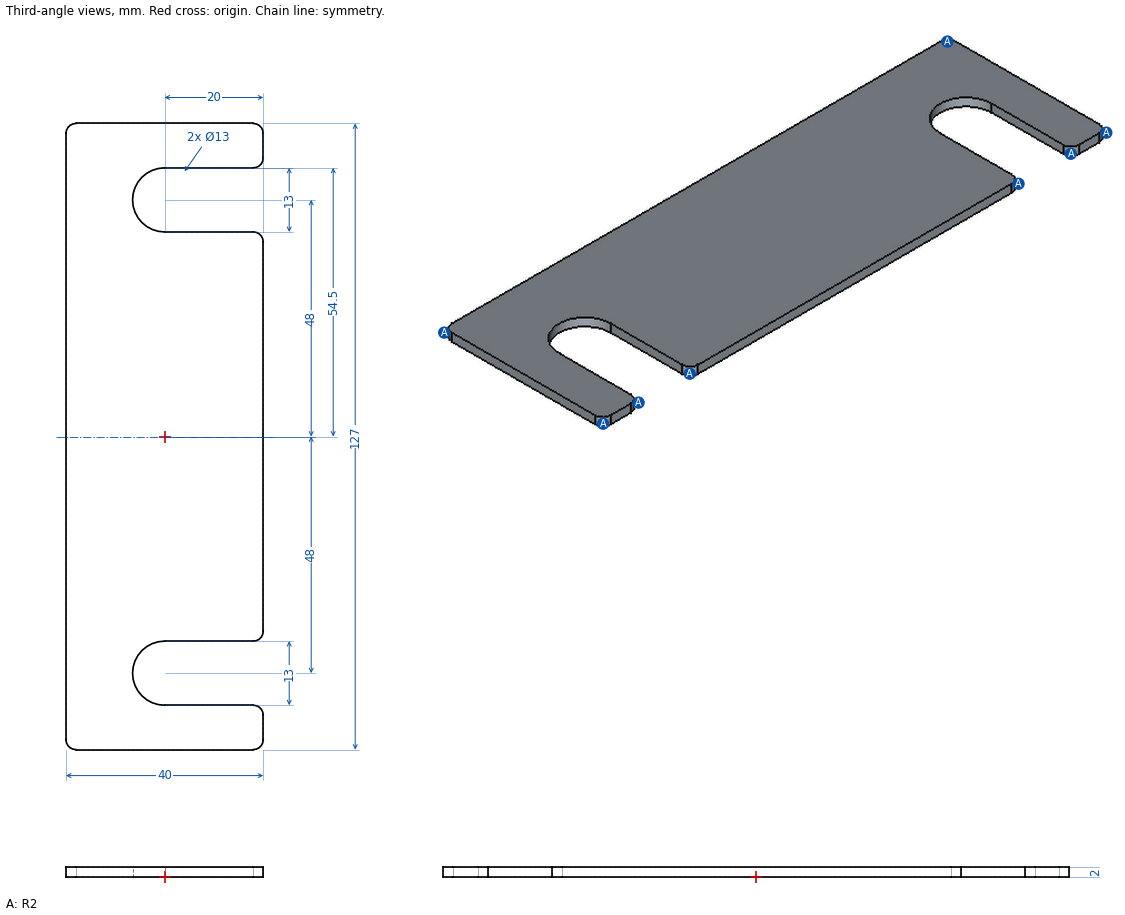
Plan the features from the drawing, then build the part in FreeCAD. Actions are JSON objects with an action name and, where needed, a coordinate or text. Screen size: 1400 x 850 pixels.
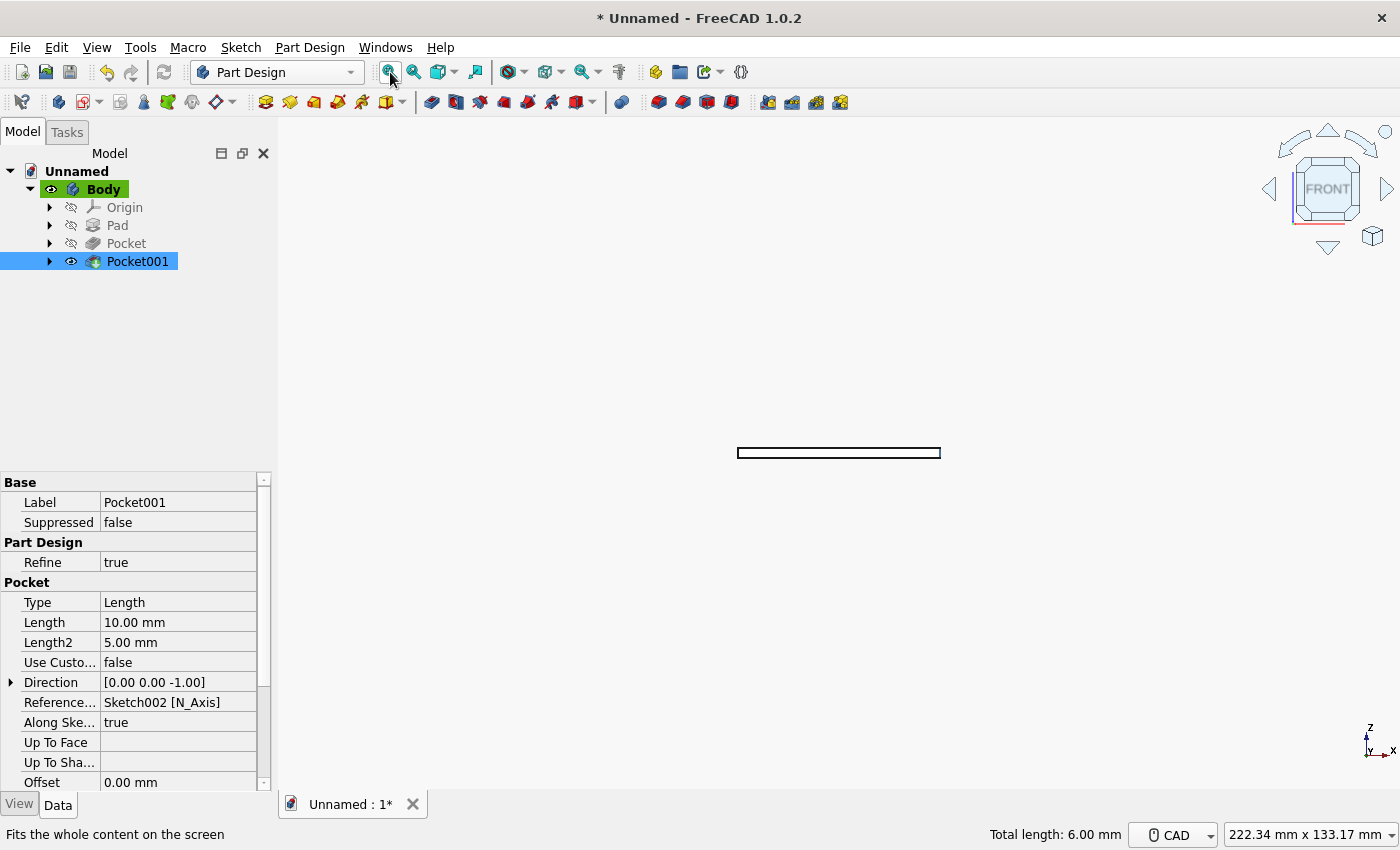
{"action": "scroll", "coordinate": [940, 452], "scroll_direction": "up", "scroll_amount": 7}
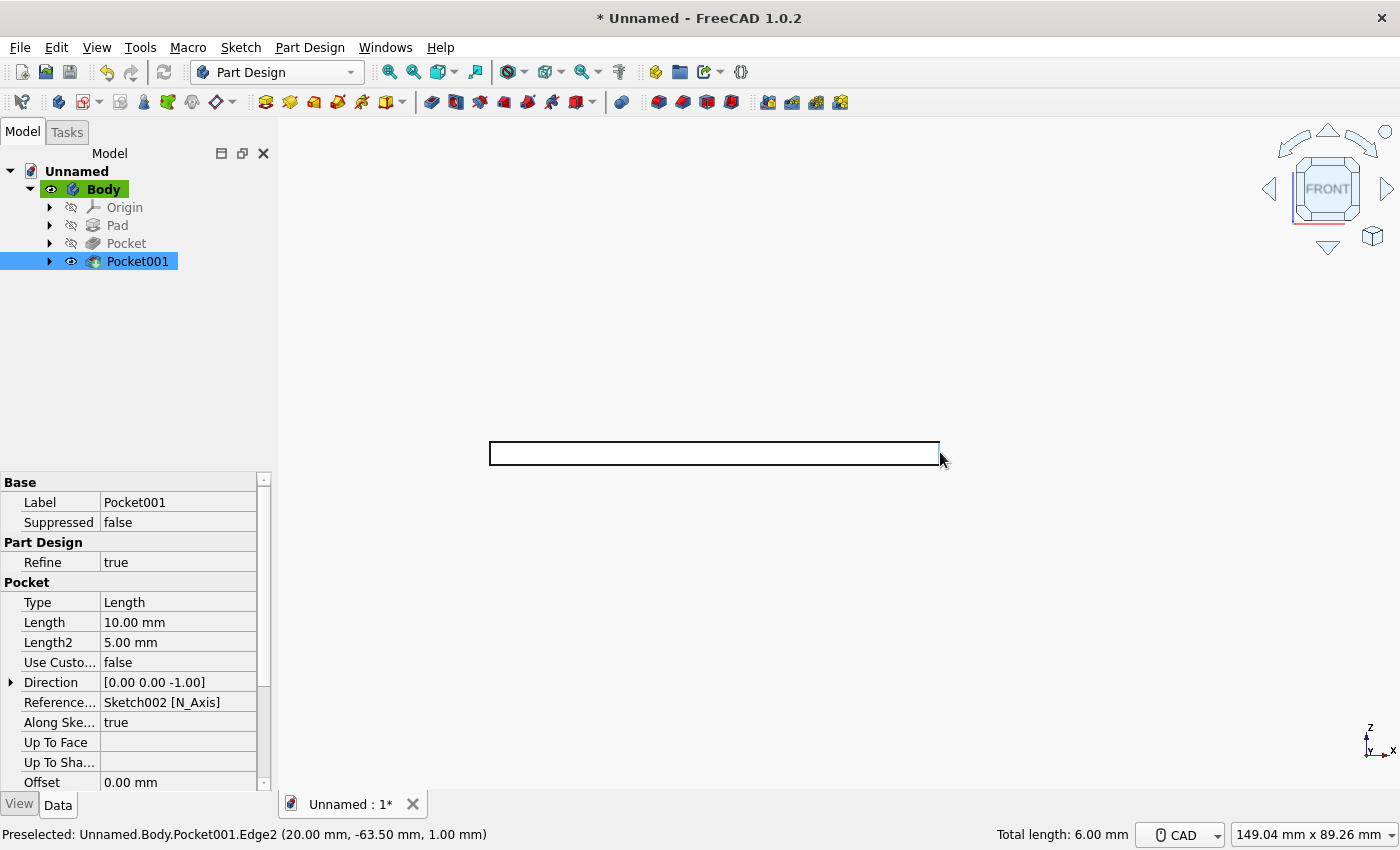
{"action": "left_click", "coordinate": [390, 72]}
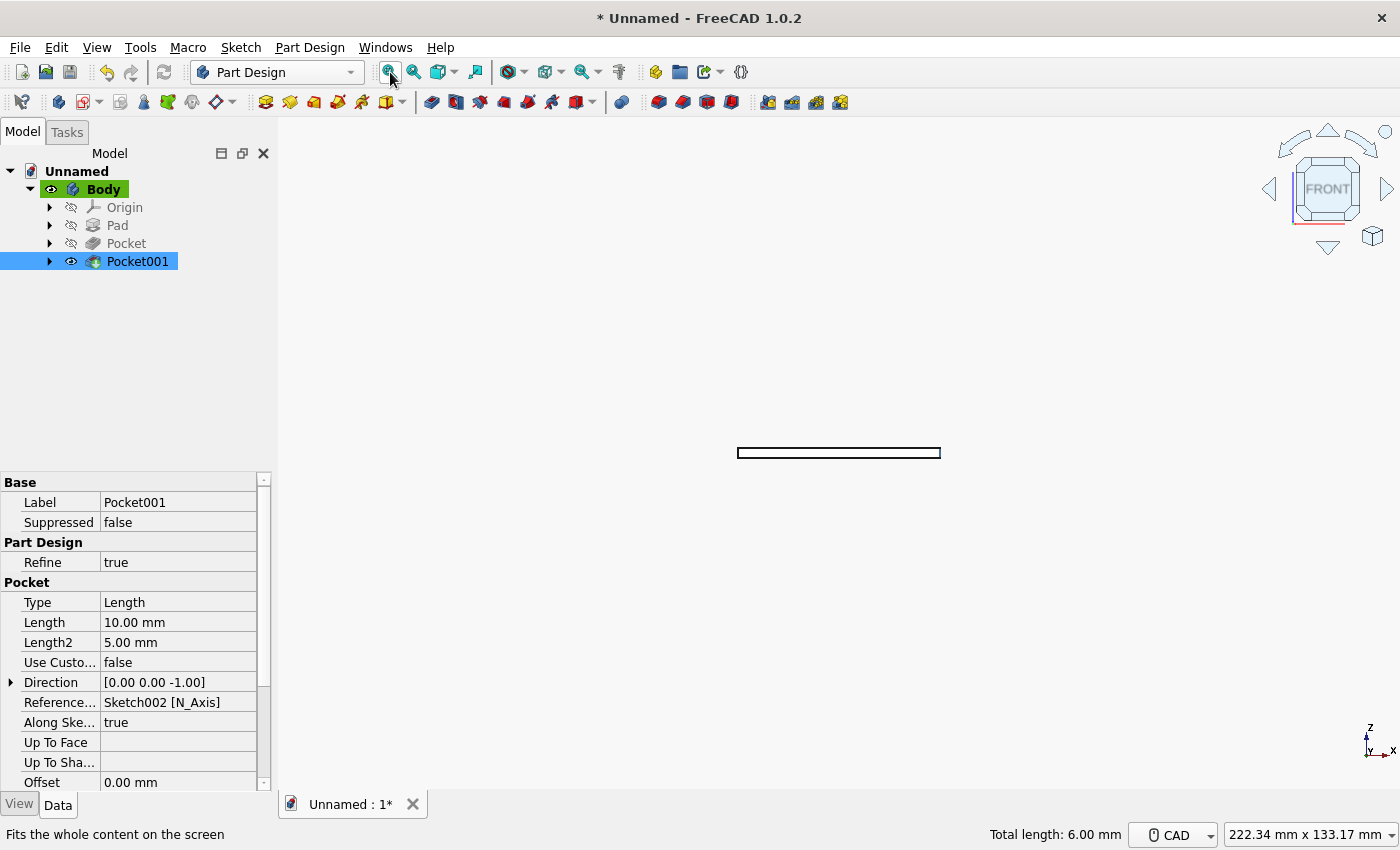
{"action": "key", "text": "3"}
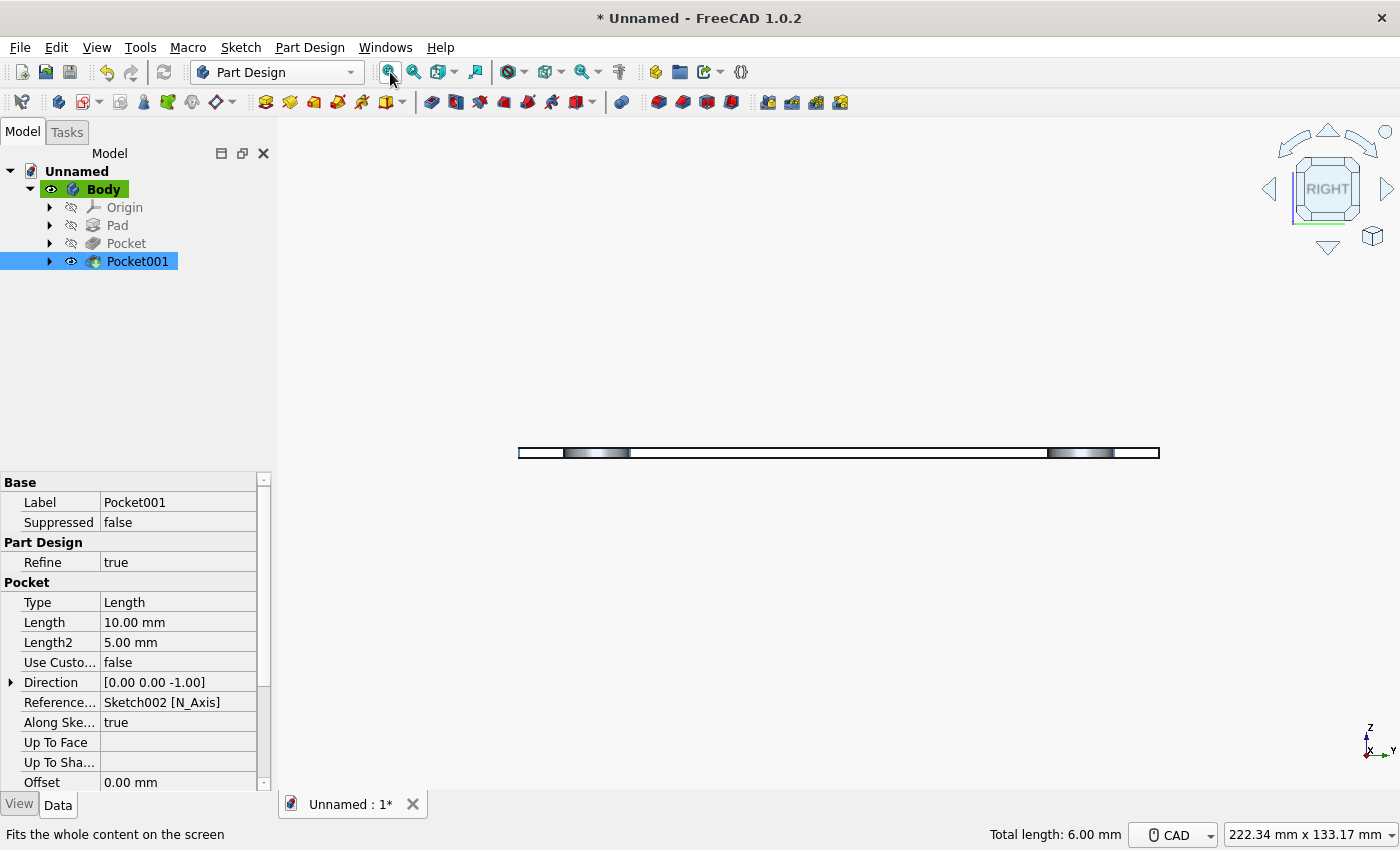
{"action": "scroll", "coordinate": [1048, 452], "scroll_direction": "up", "scroll_amount": 7}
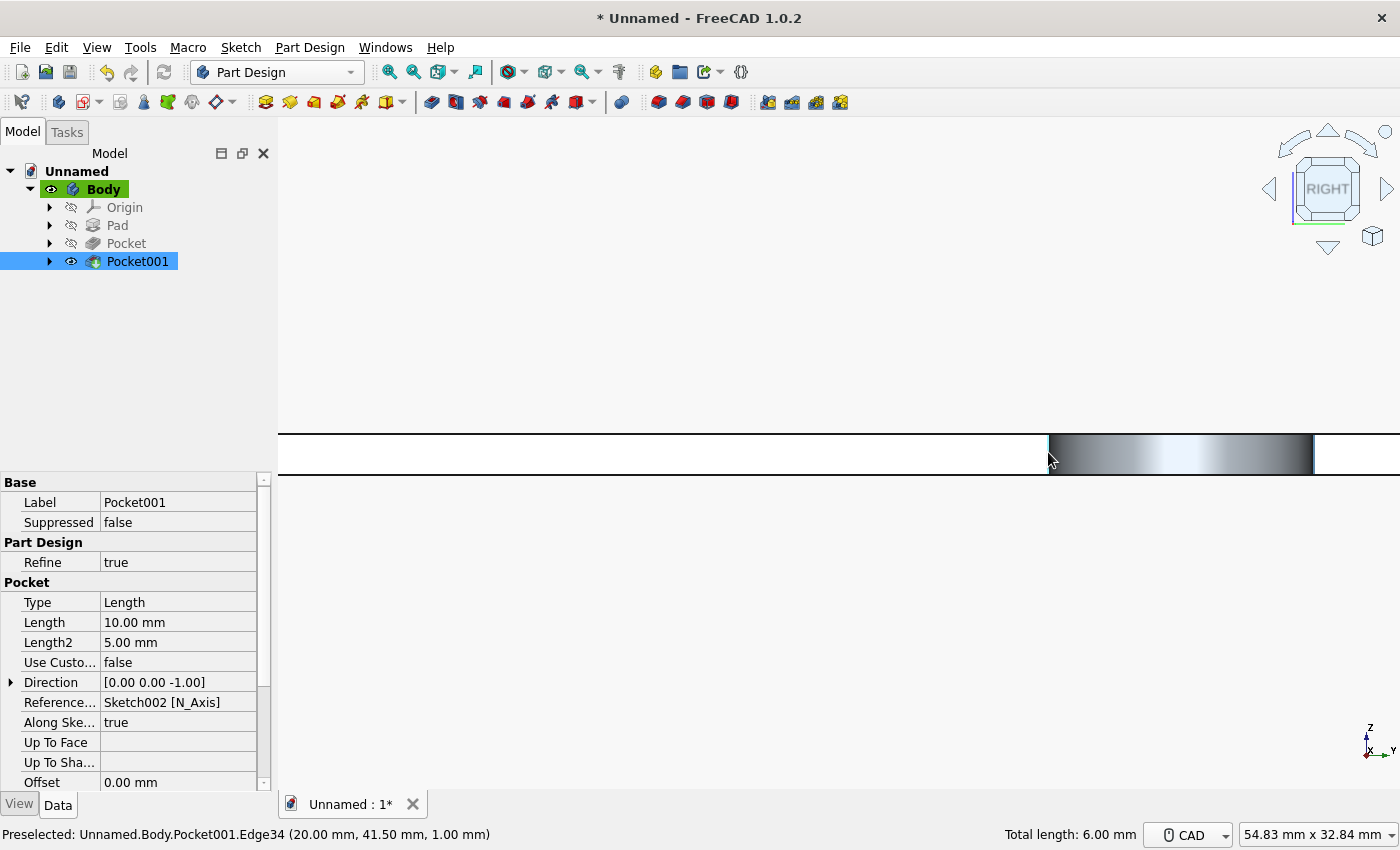
{"action": "left_click", "coordinate": [1048, 454], "text": "ctrl"}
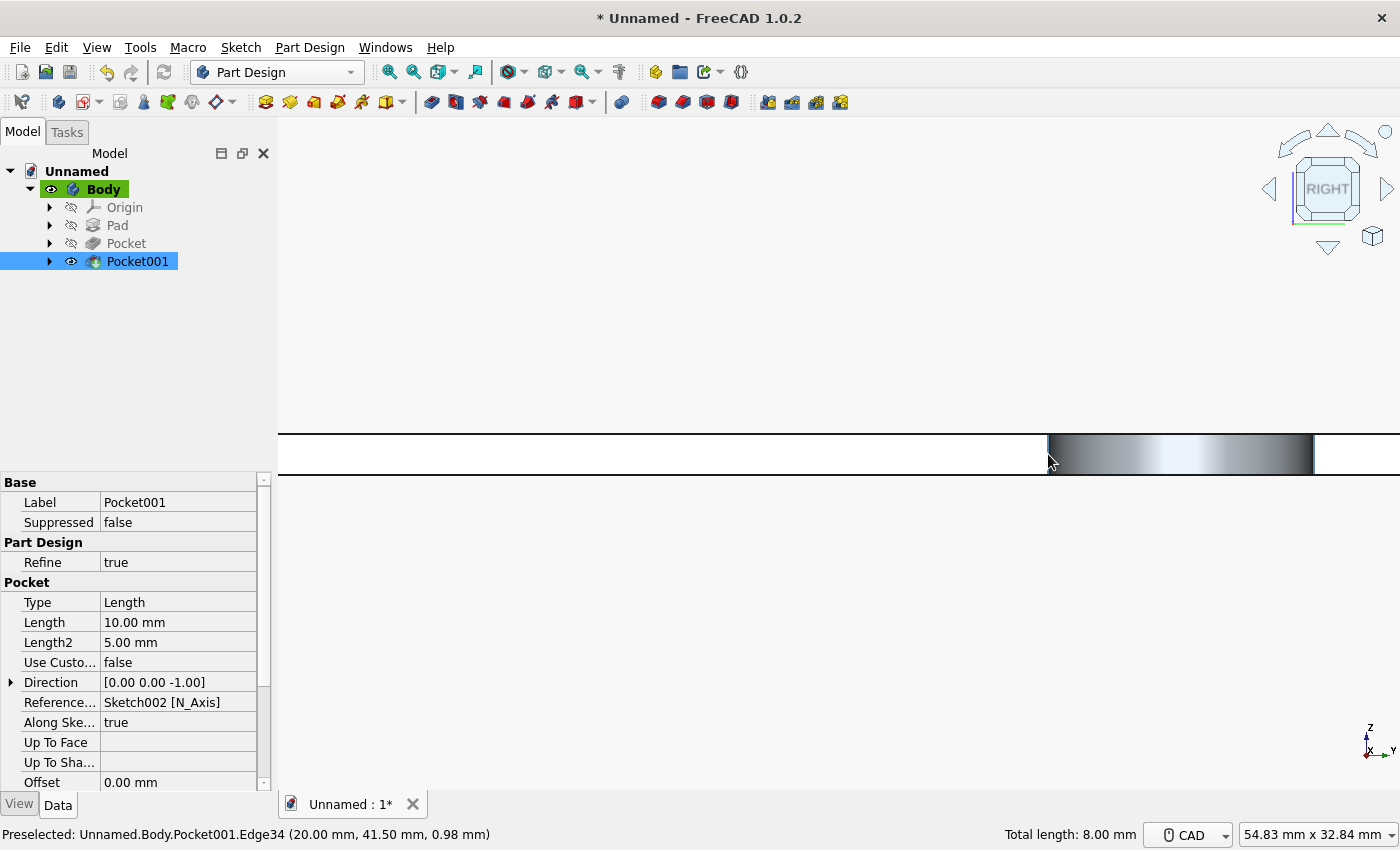
{"action": "left_click", "coordinate": [390, 72]}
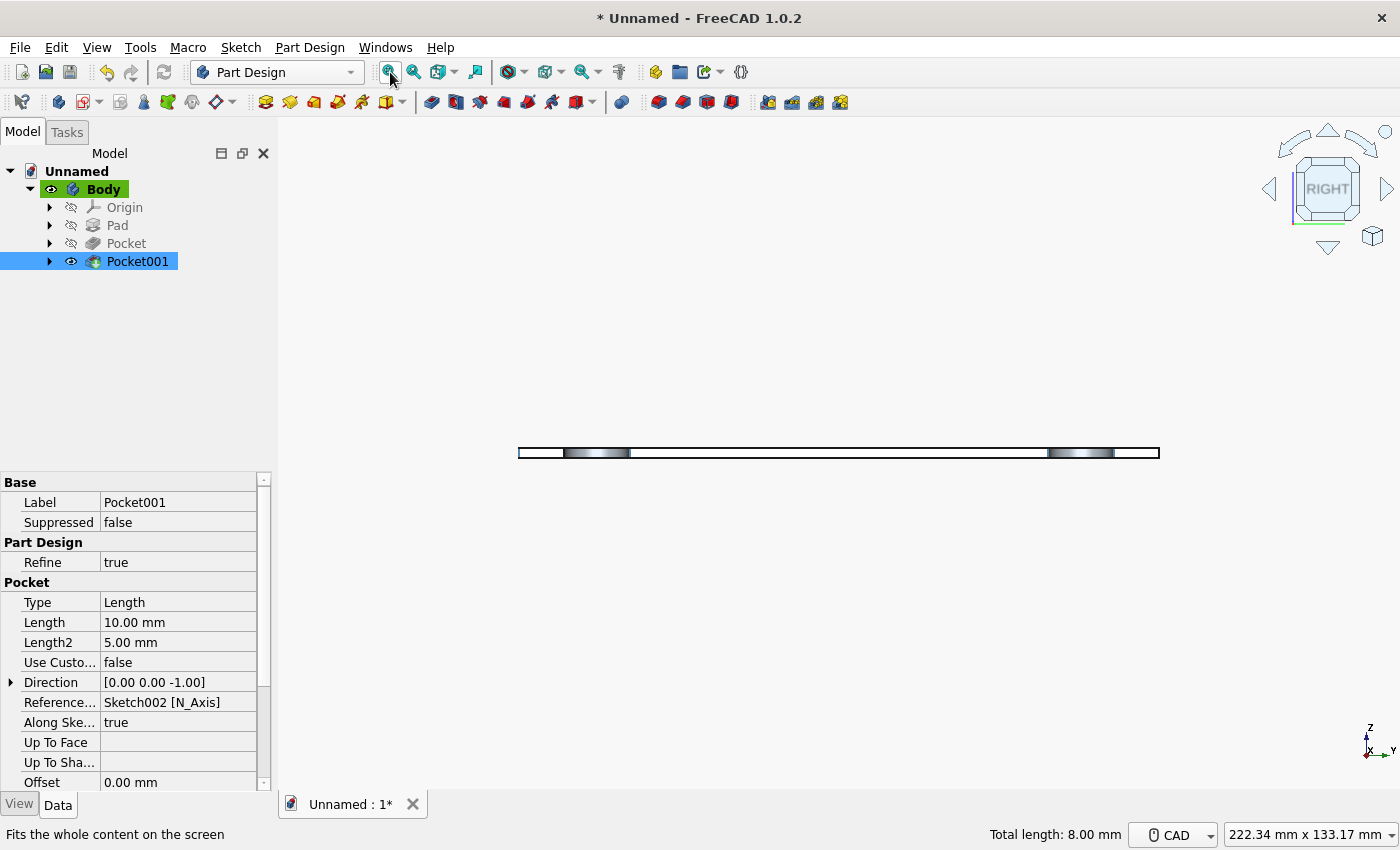
{"action": "key", "text": "5"}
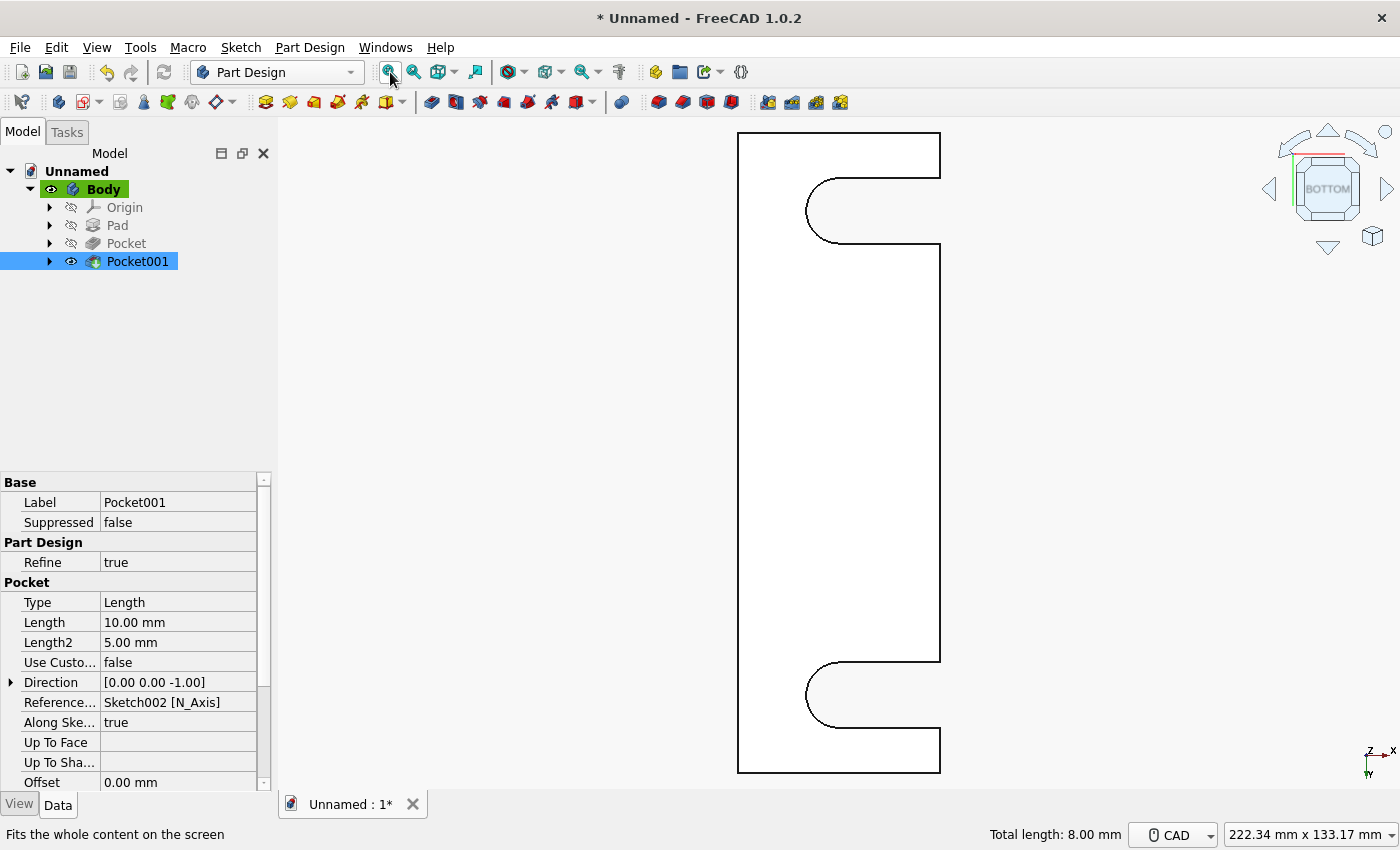
{"action": "scroll", "coordinate": [940, 177], "scroll_direction": "up", "scroll_amount": 7}